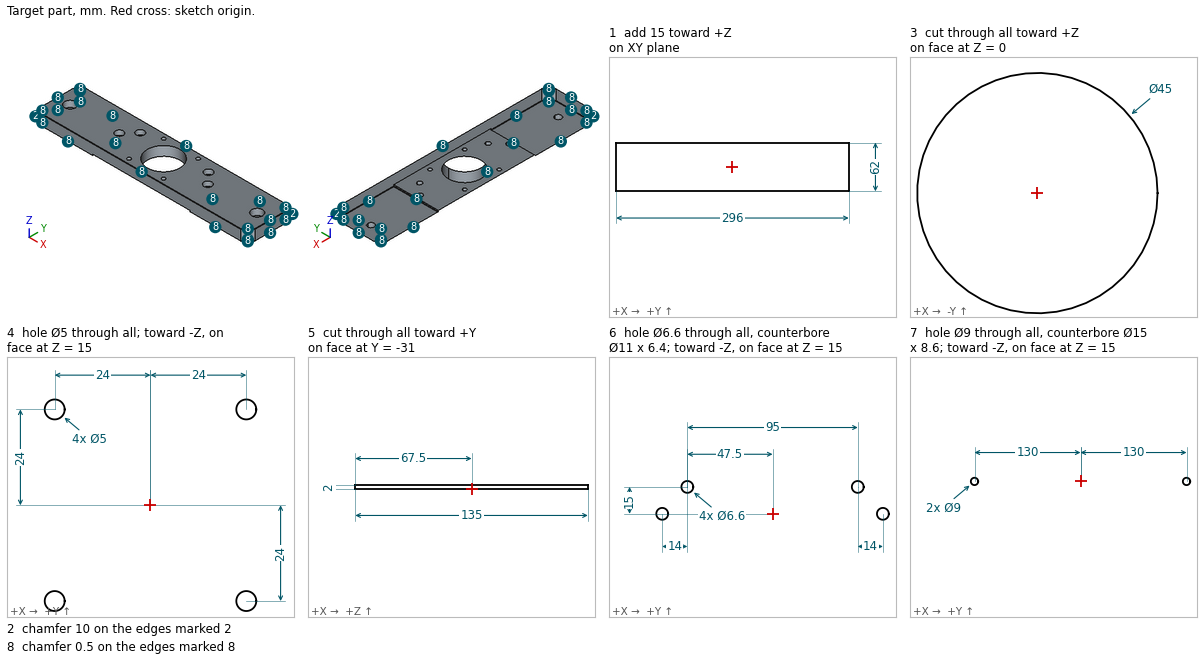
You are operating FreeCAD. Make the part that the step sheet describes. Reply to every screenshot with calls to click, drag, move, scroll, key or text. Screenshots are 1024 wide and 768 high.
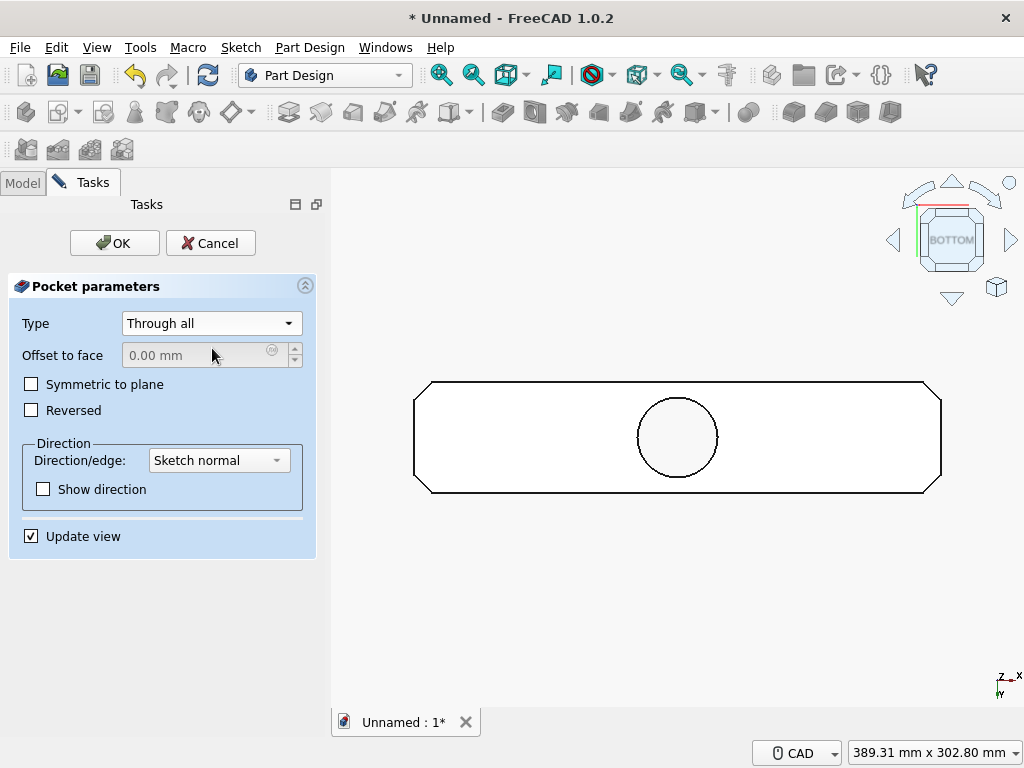
click(115, 243)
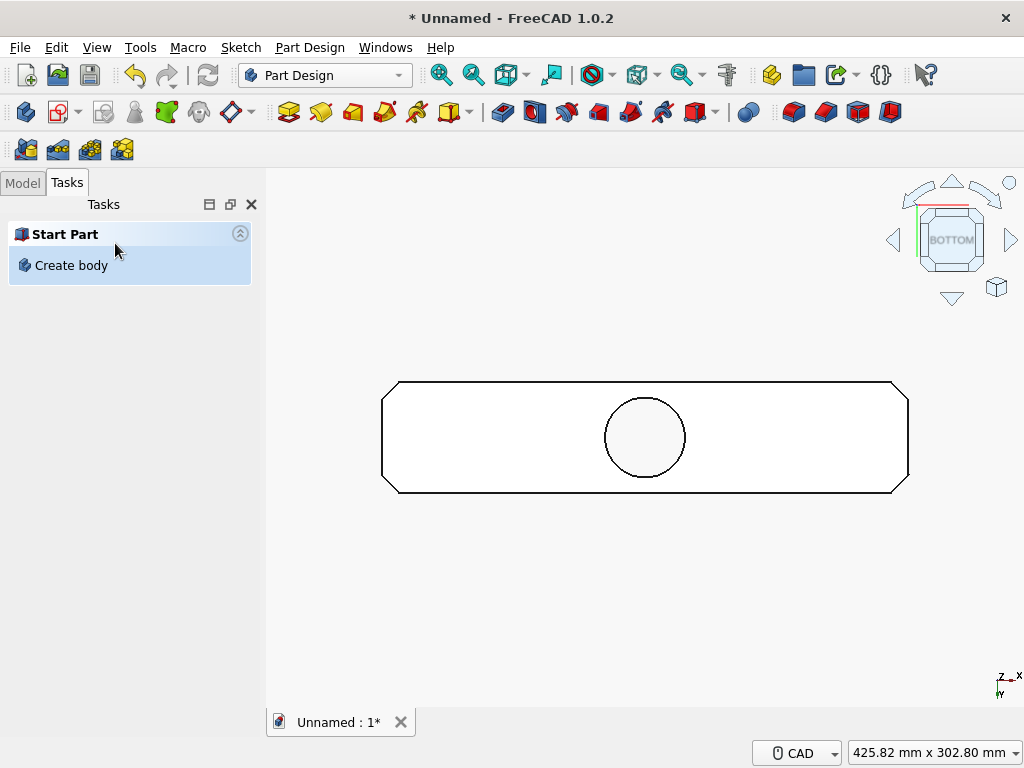
key(0)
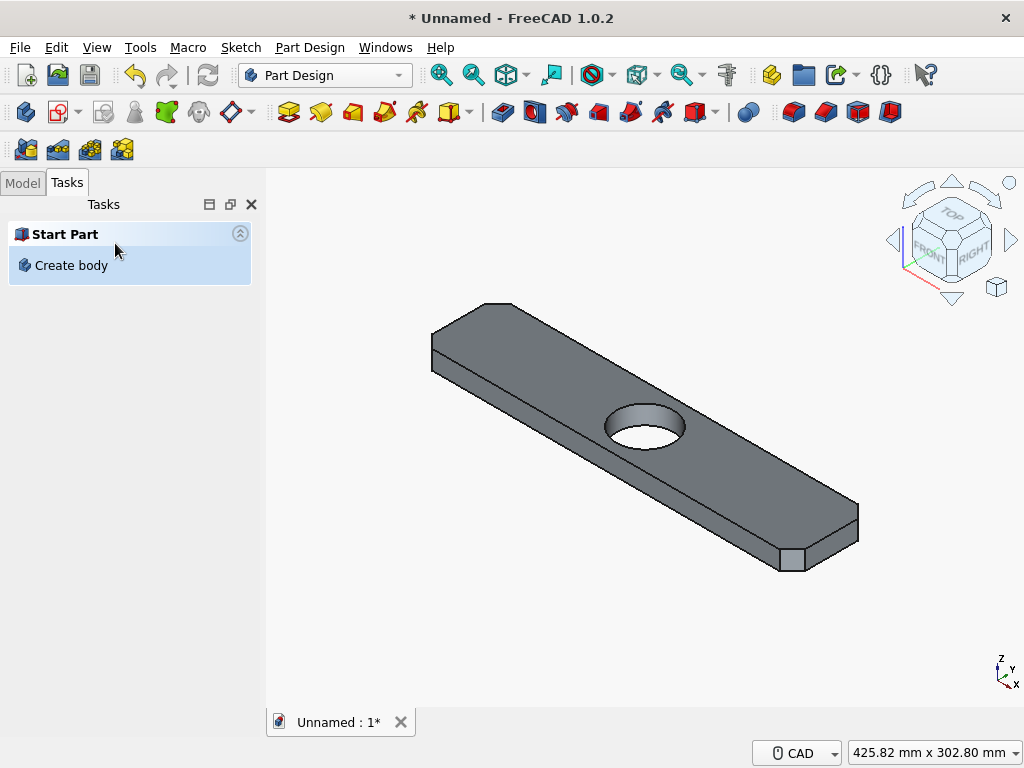
click(751, 487)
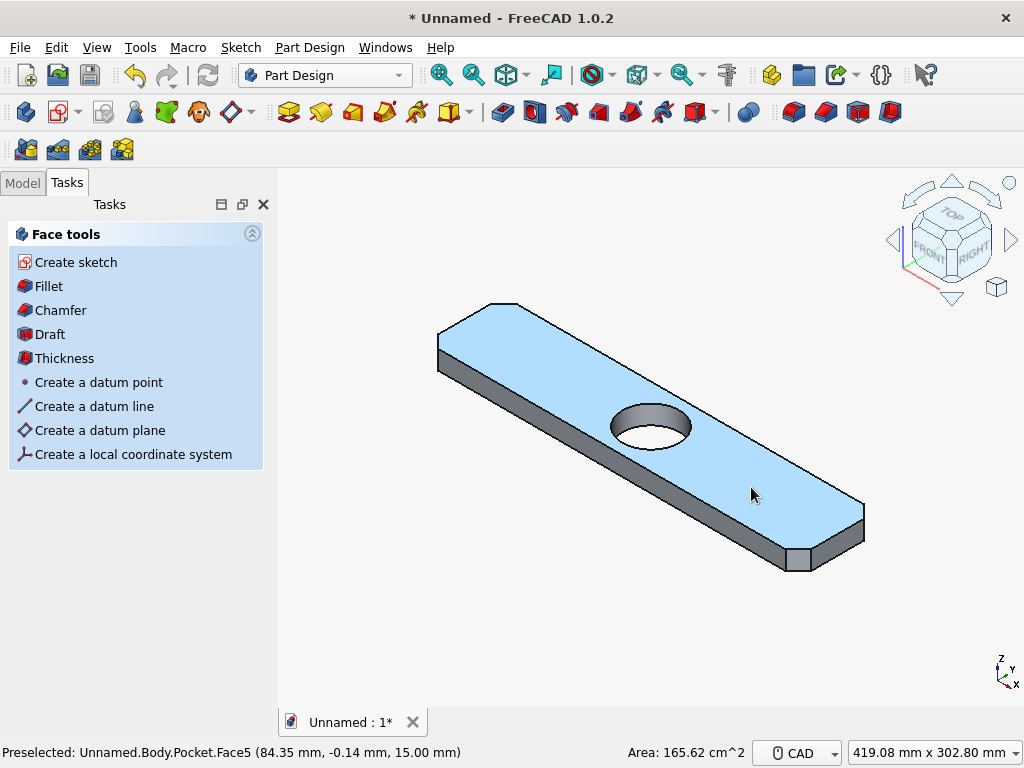
click(58, 112)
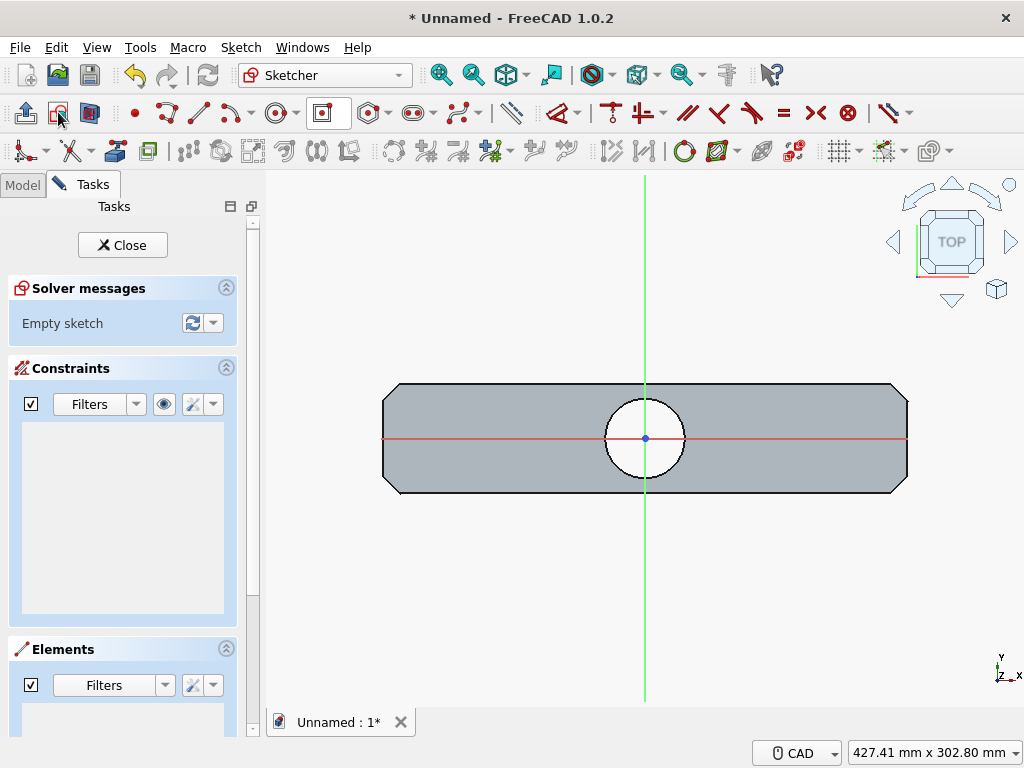
scroll(675, 438, up, 6)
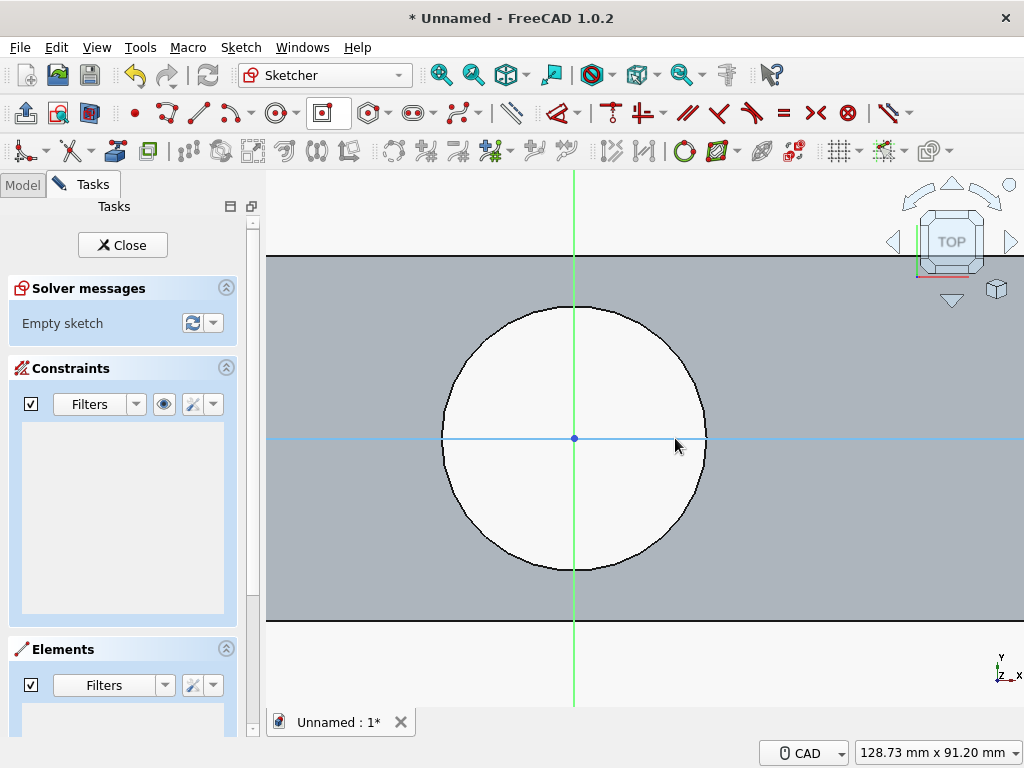
click(276, 114)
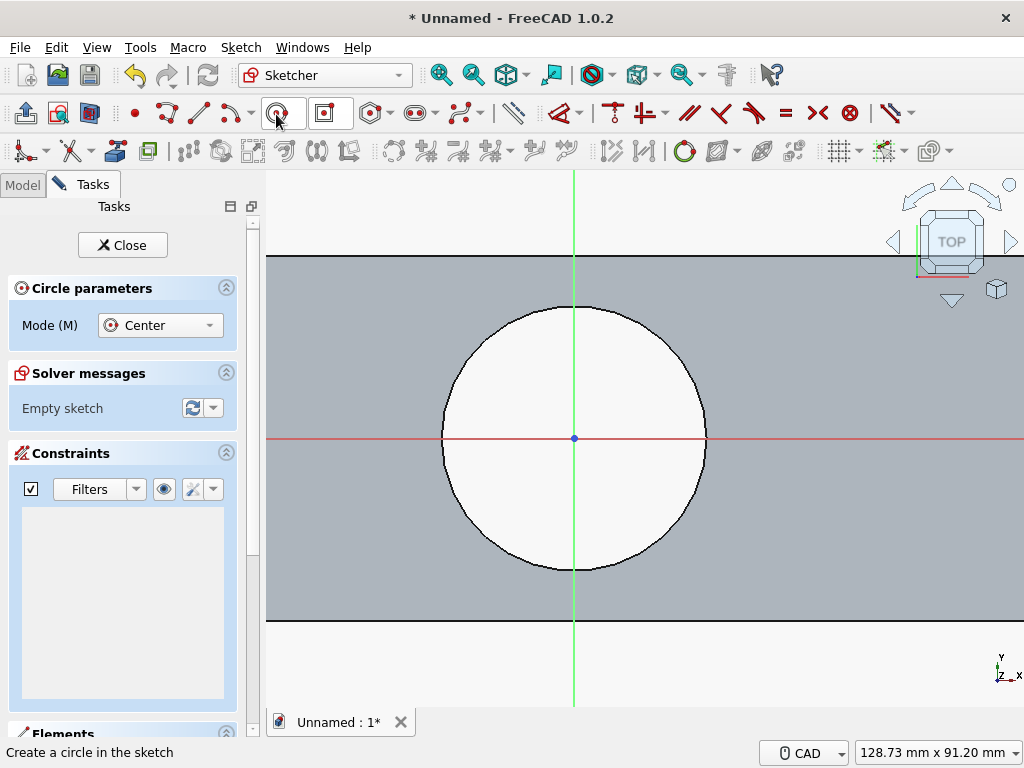
scroll(433, 297, up, 3)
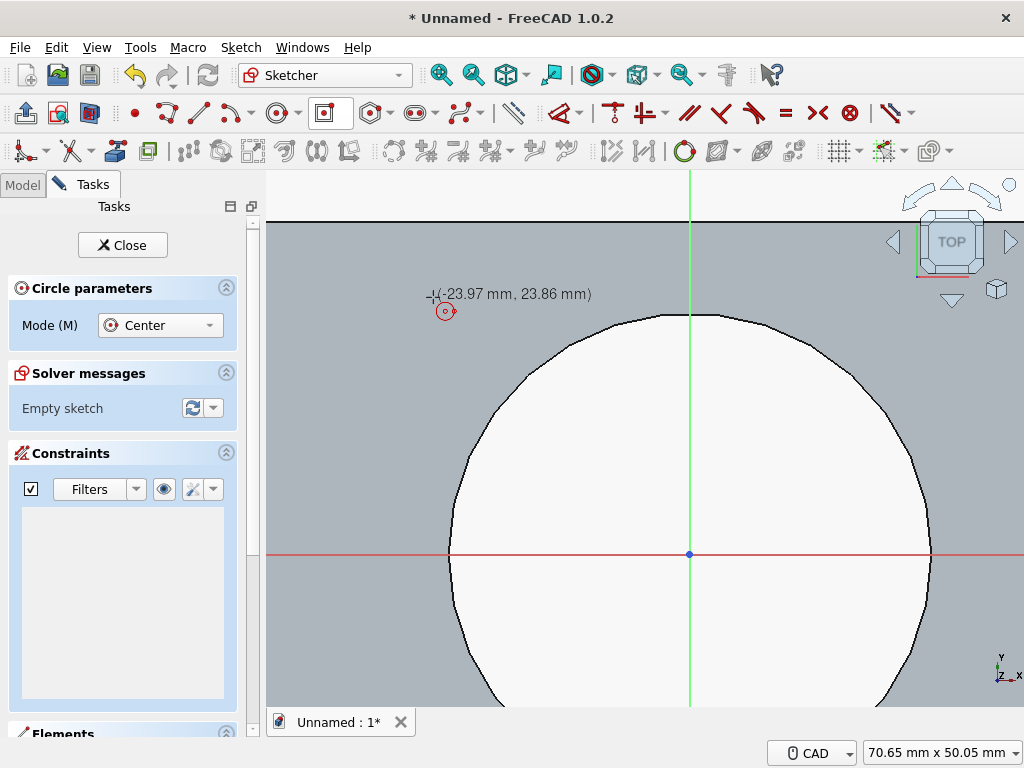
click(433, 297)
move(451, 278)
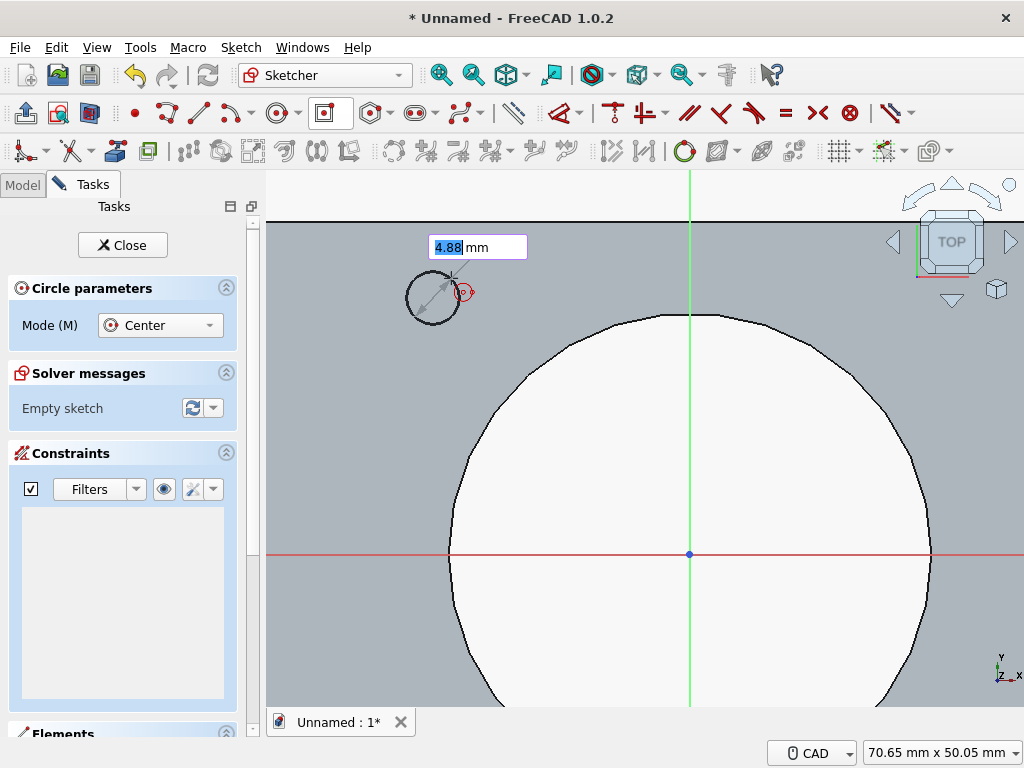
text(5)
key(Return)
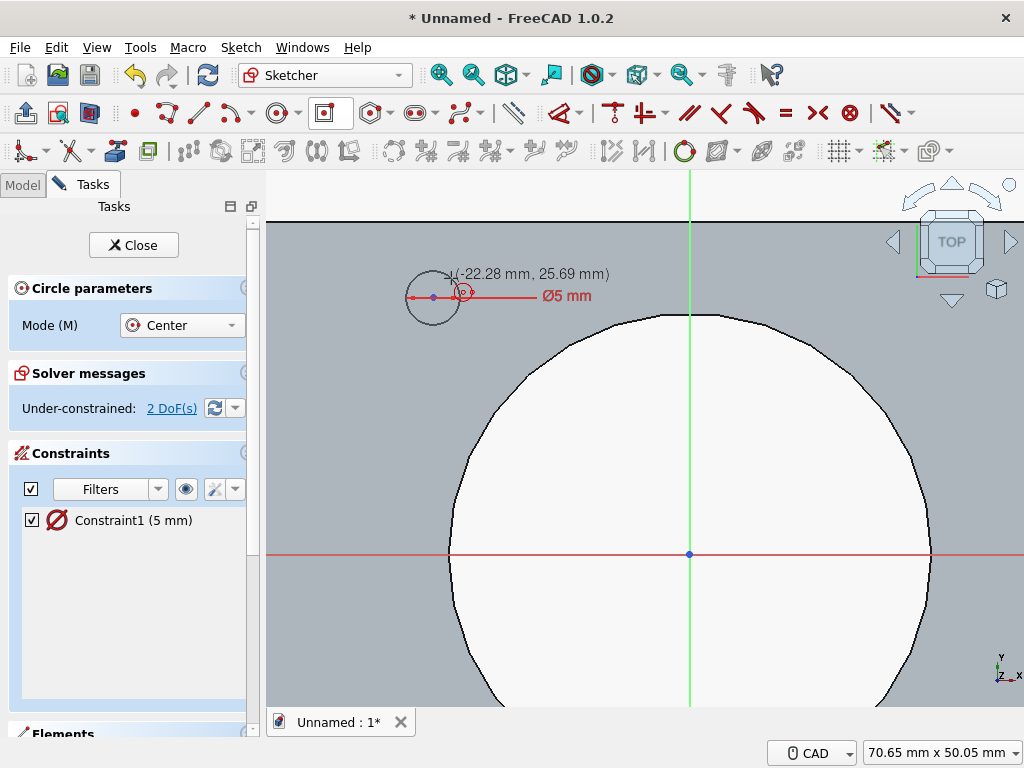
scroll(438, 297, down, 3)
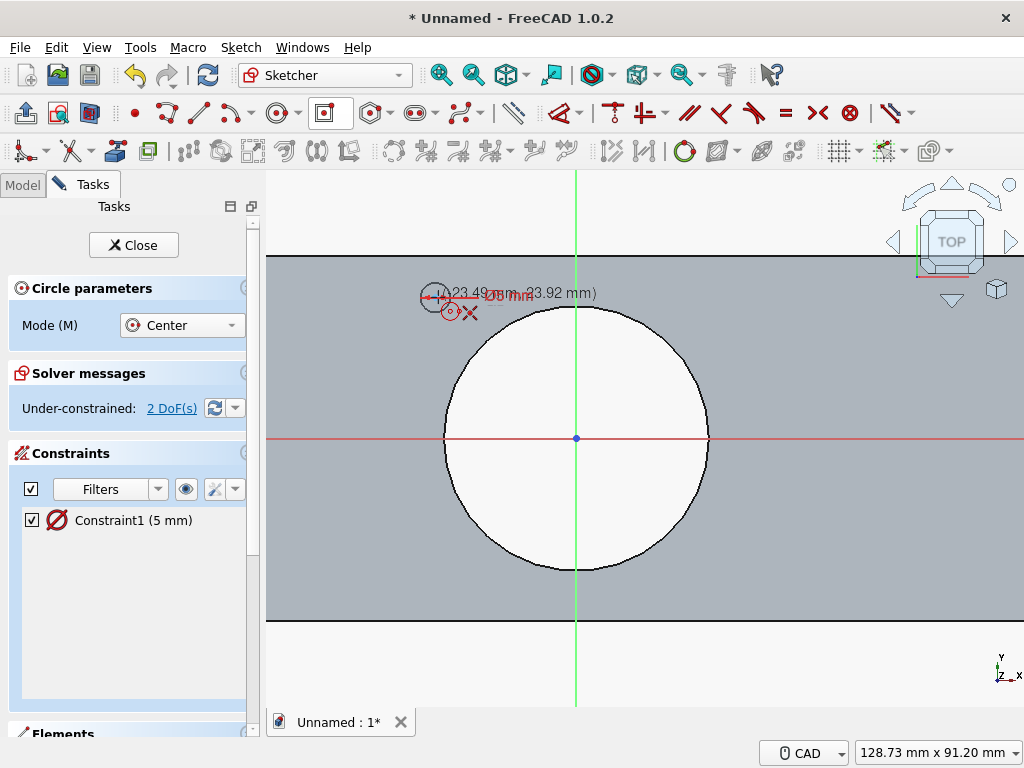
scroll(718, 297, up, 3)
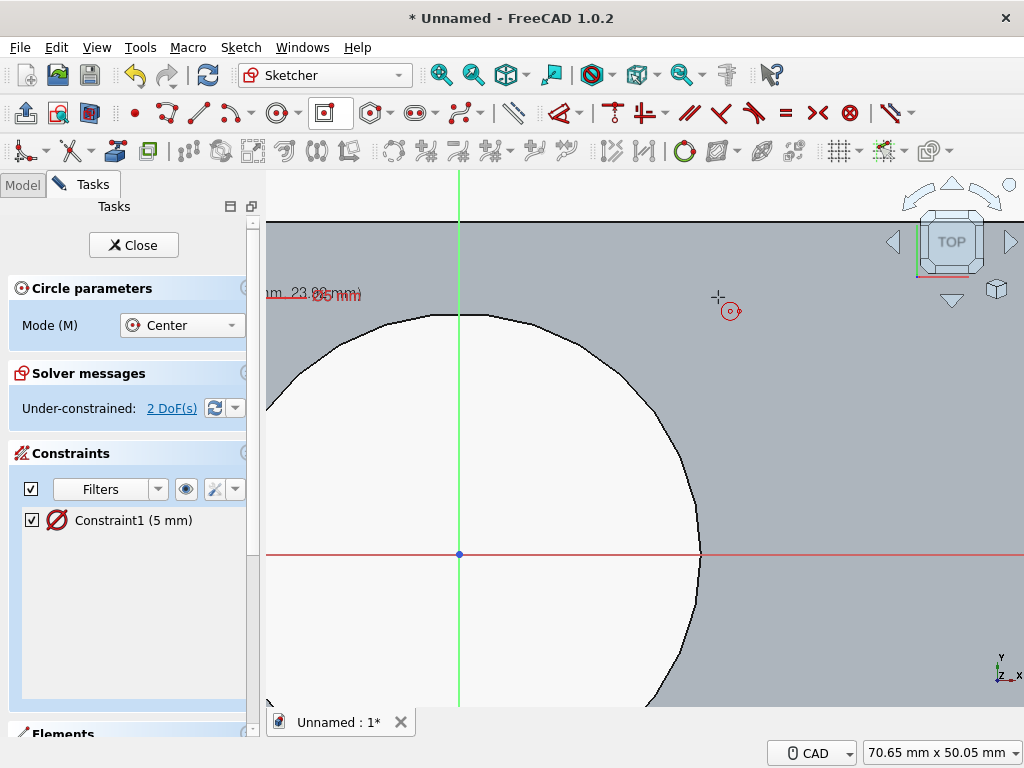
click(717, 297)
move(736, 278)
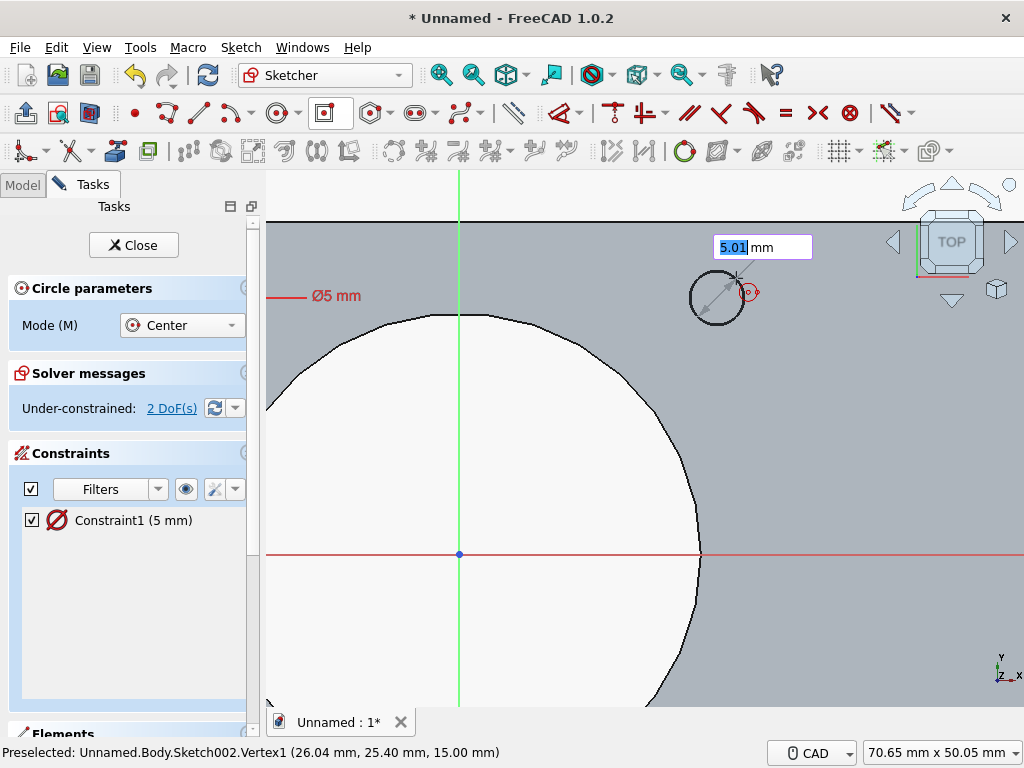
text(5)
key(Return)